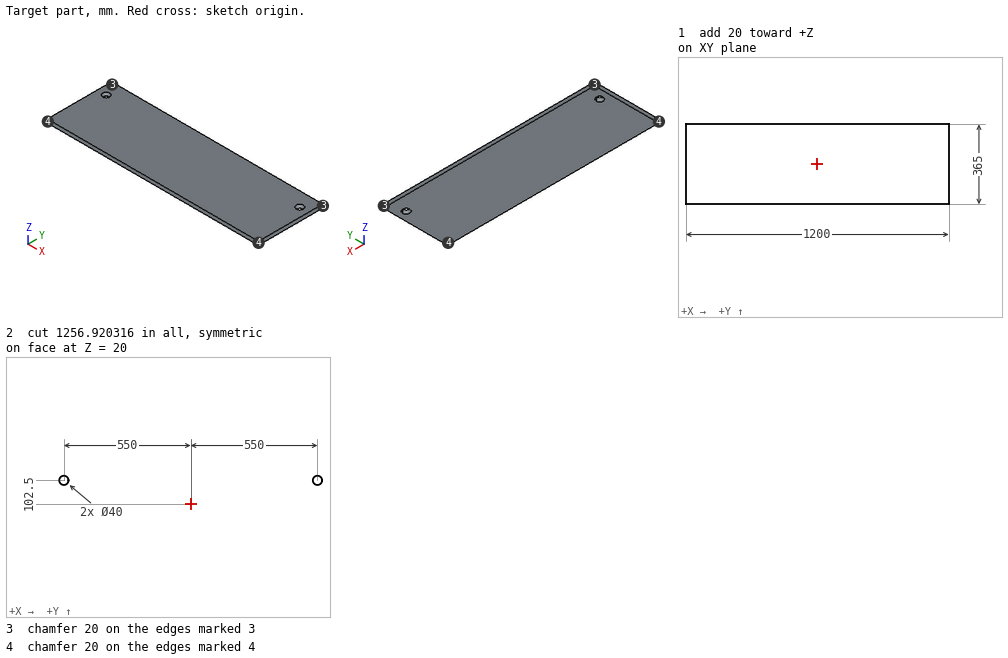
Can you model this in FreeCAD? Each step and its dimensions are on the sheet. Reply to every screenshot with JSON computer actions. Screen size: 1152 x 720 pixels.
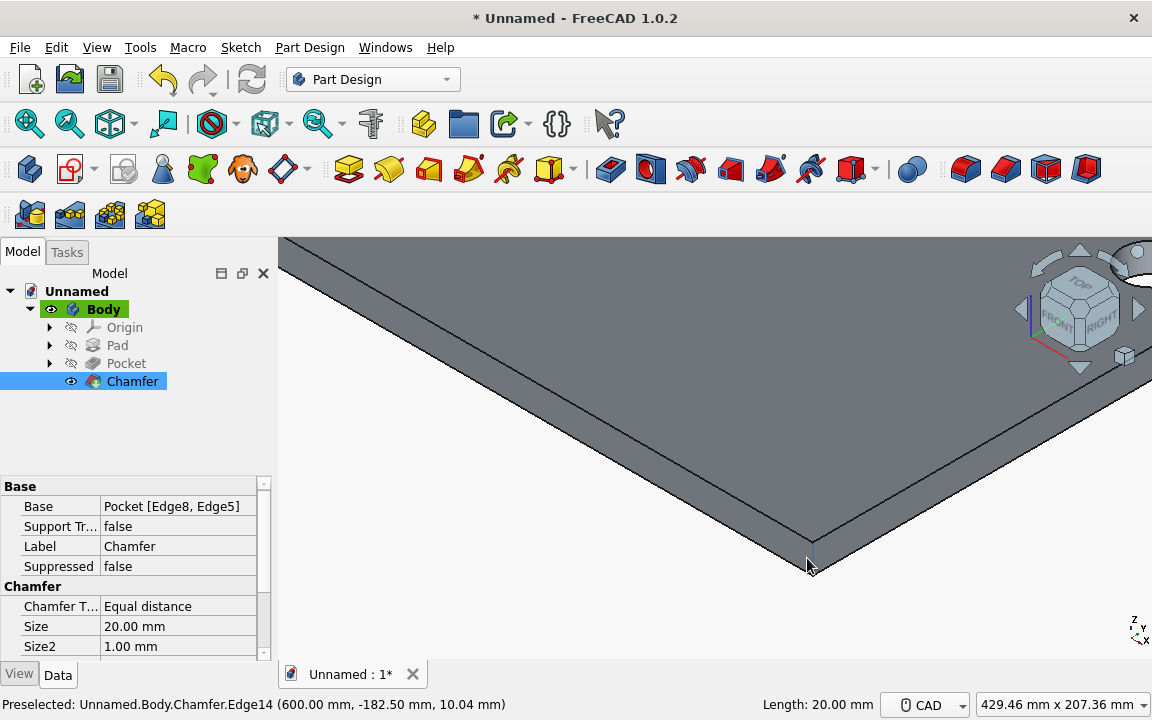
{"action": "key", "text": "v f"}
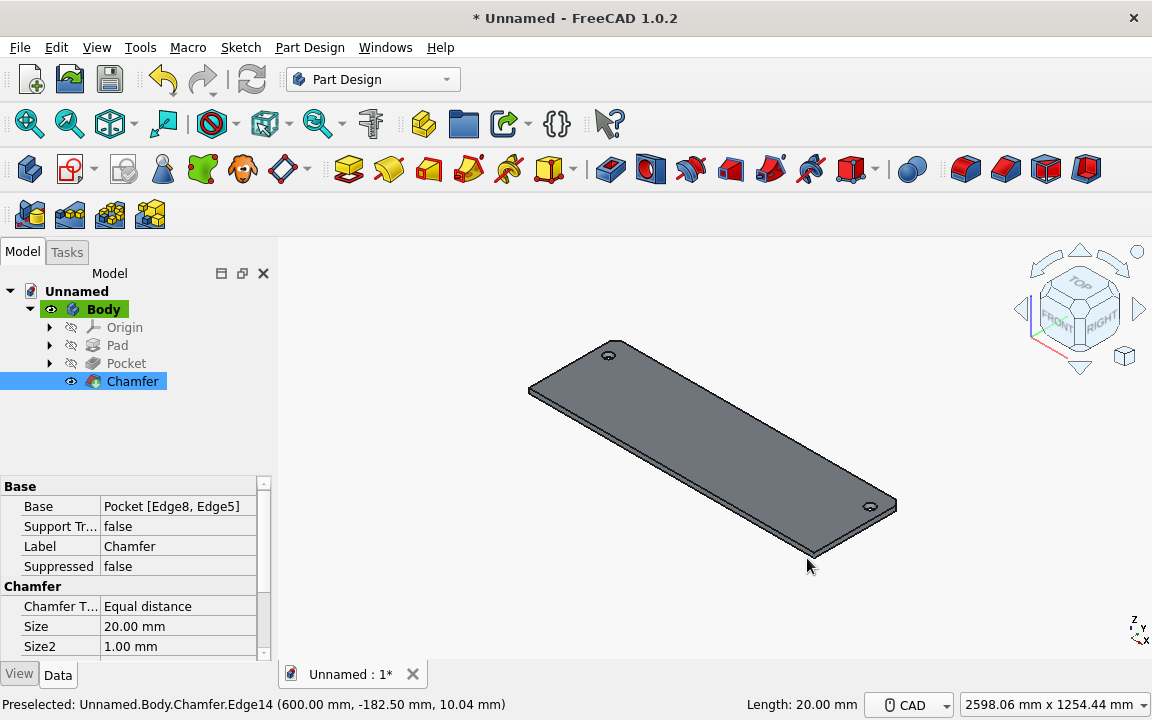
{"action": "key", "text": "2"}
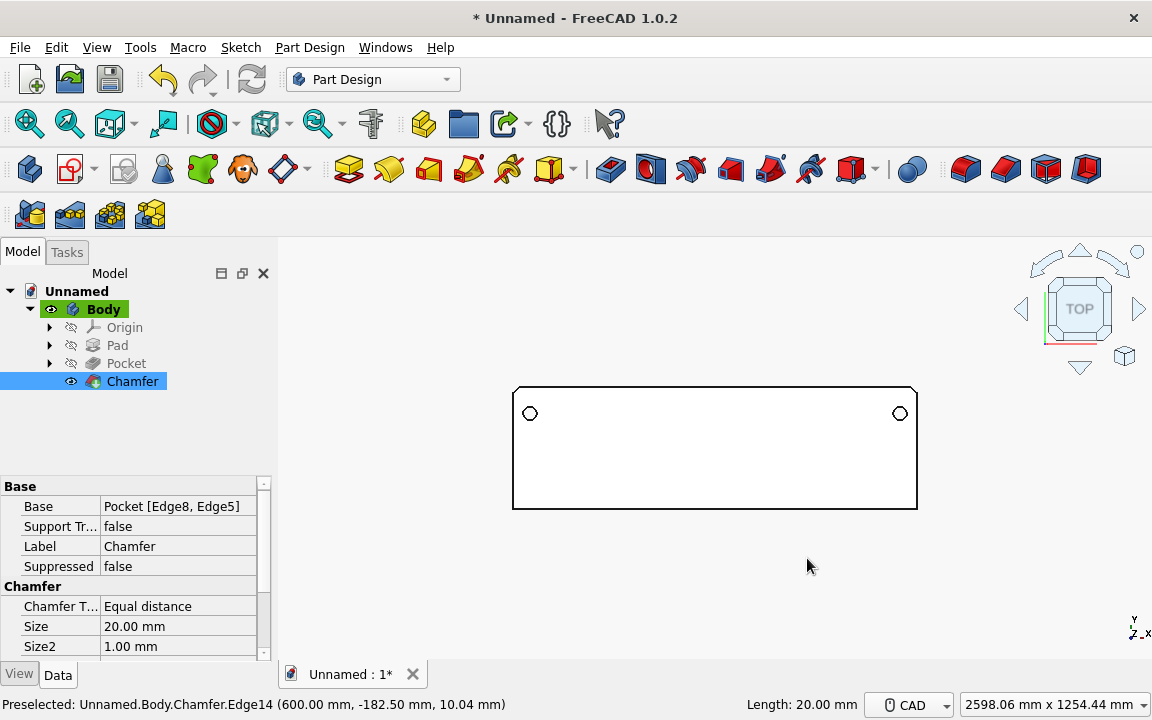
{"action": "scroll", "coordinate": [513, 508], "scroll_direction": "up", "scroll_amount": 9}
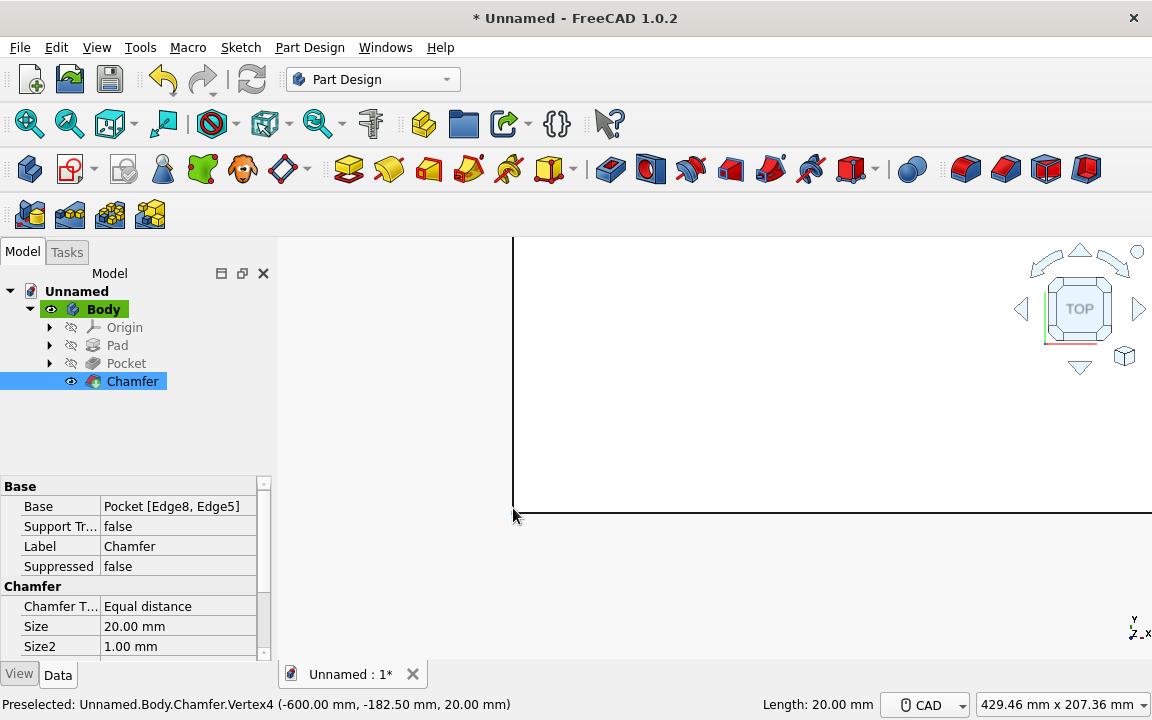
{"action": "left_click", "coordinate": [30, 124]}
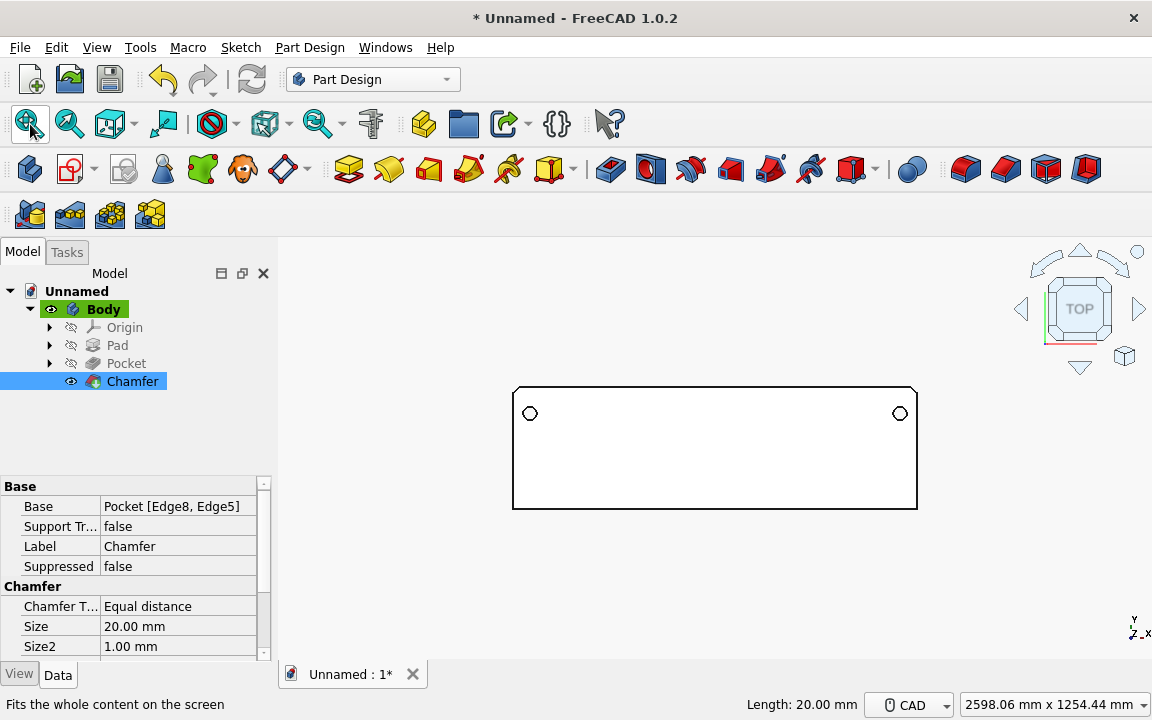
{"action": "key", "text": "1"}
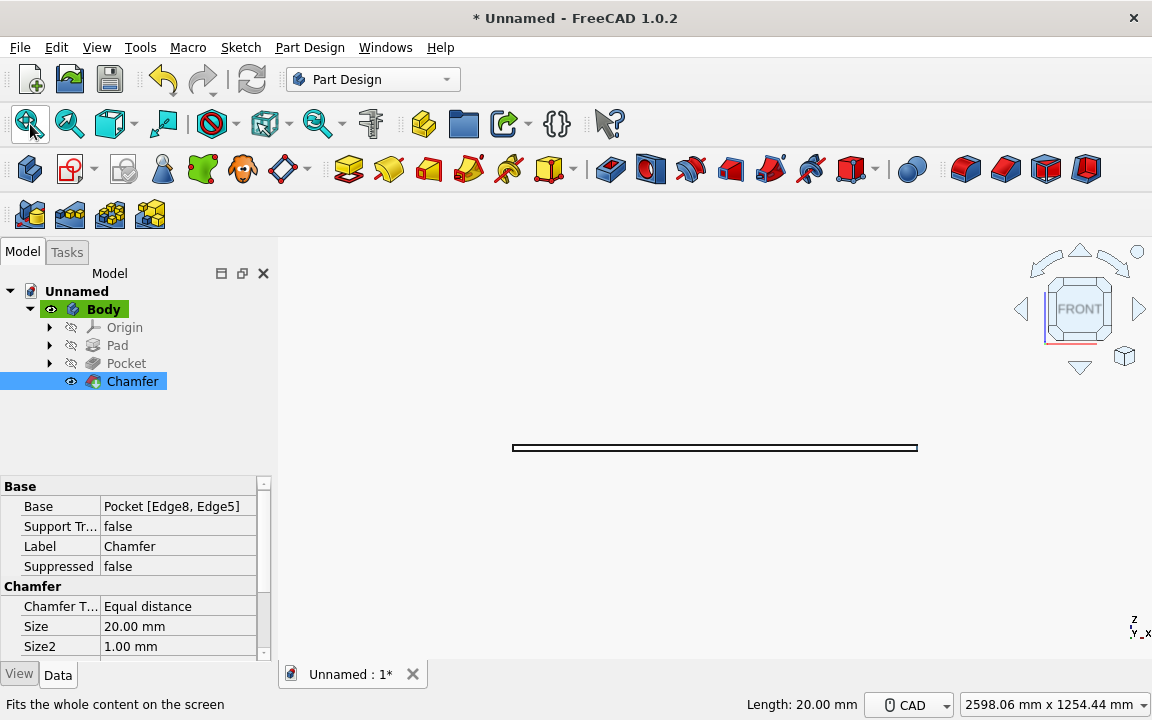
{"action": "scroll", "coordinate": [513, 447], "scroll_direction": "up", "scroll_amount": 9}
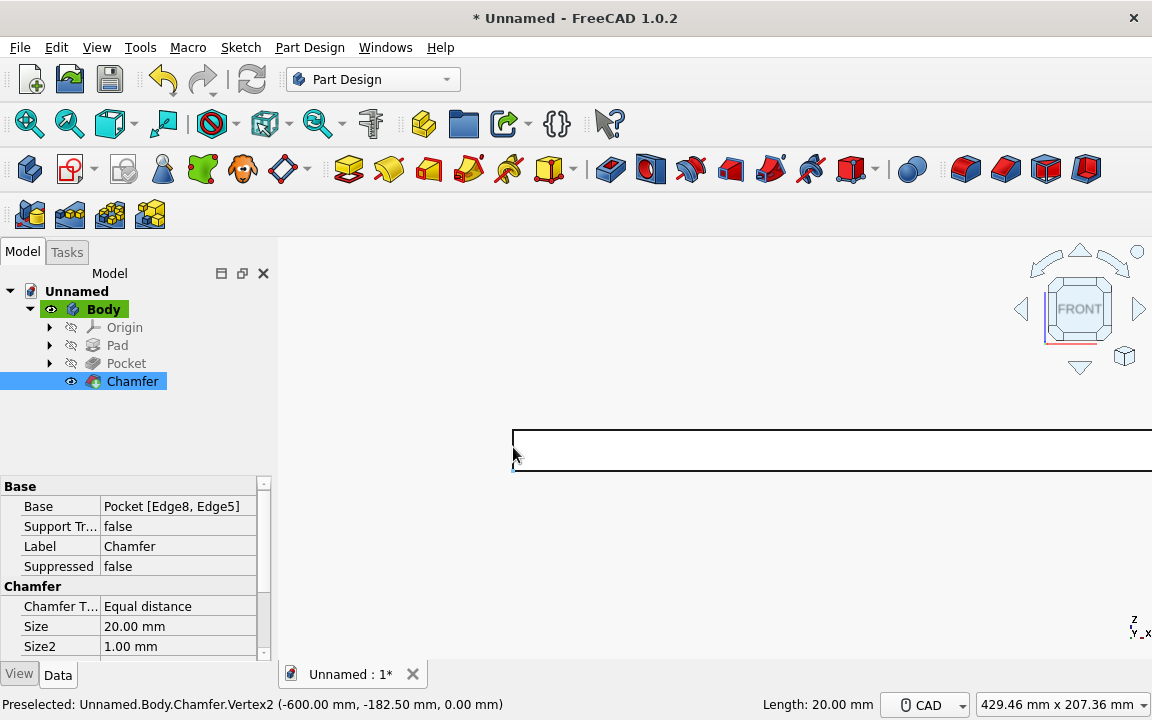
{"action": "left_click", "coordinate": [513, 450], "text": "ctrl"}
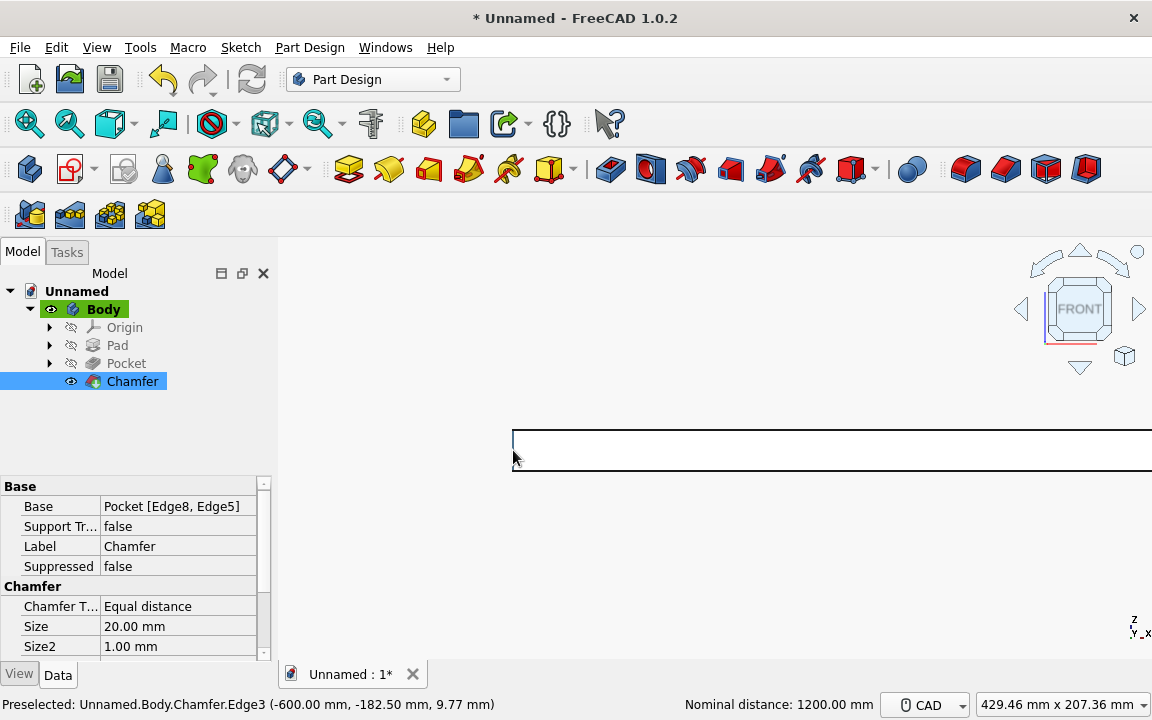
{"action": "left_click", "coordinate": [1006, 170]}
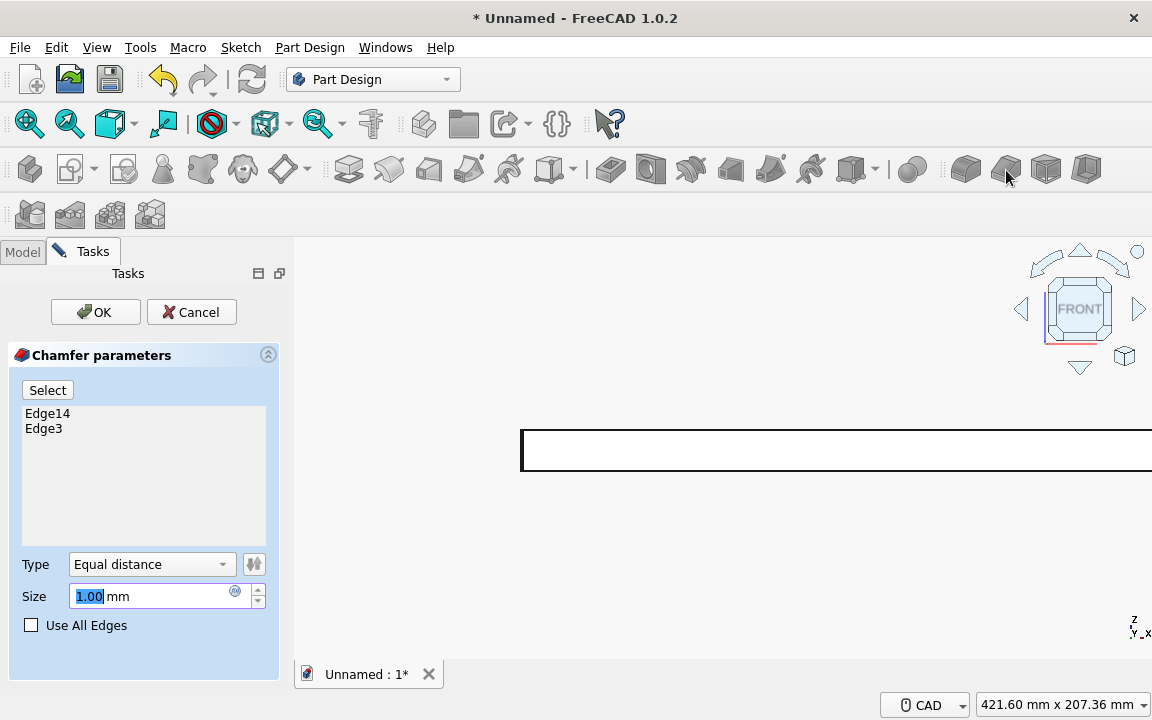
{"action": "type", "text": "20"}
{"action": "key", "text": "Tab"}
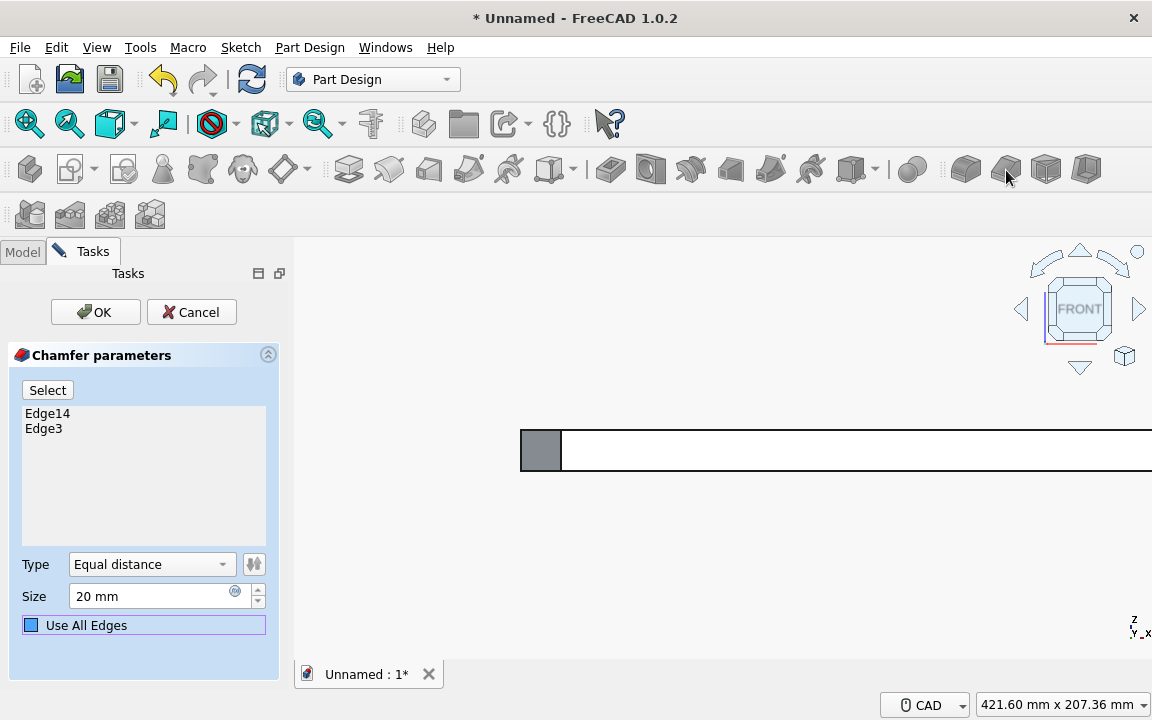
{"action": "left_click", "coordinate": [96, 312]}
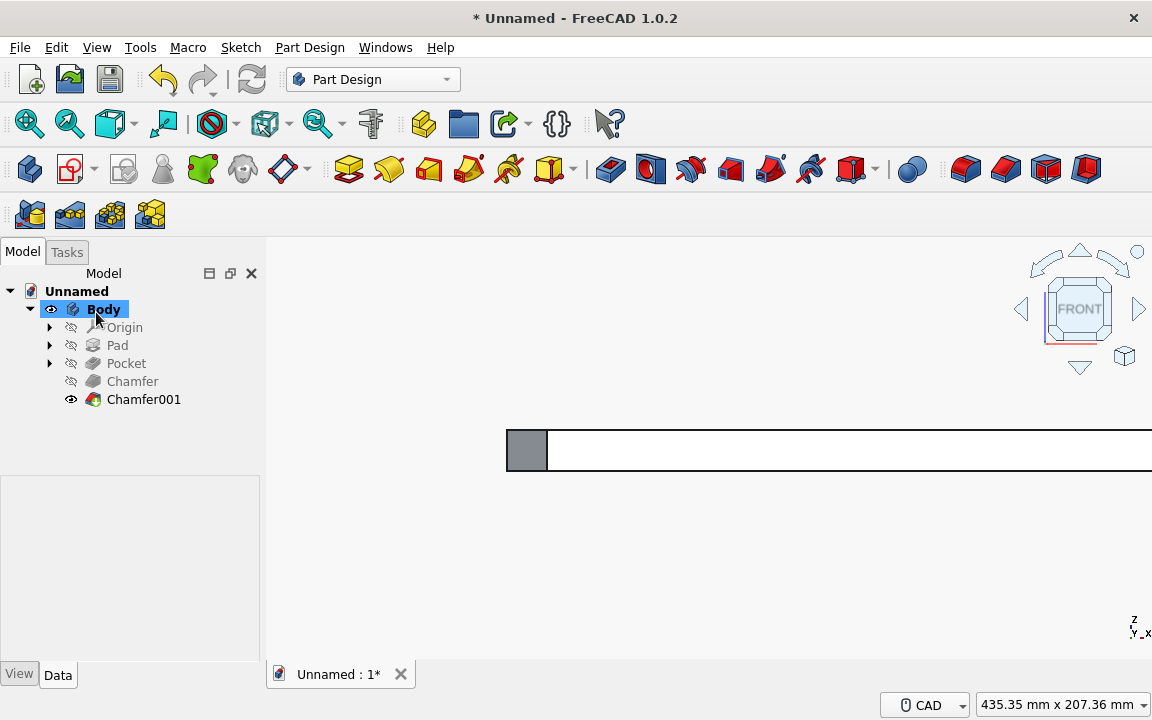
{"action": "key", "text": "0"}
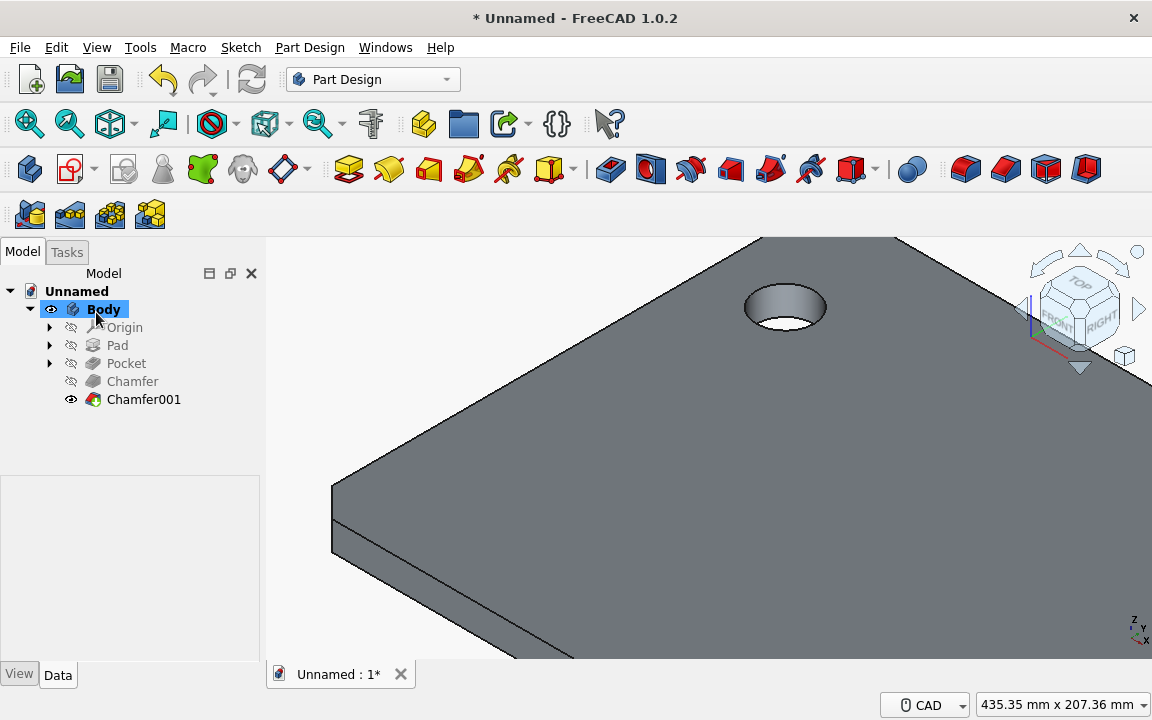
{"action": "key", "text": "v f"}